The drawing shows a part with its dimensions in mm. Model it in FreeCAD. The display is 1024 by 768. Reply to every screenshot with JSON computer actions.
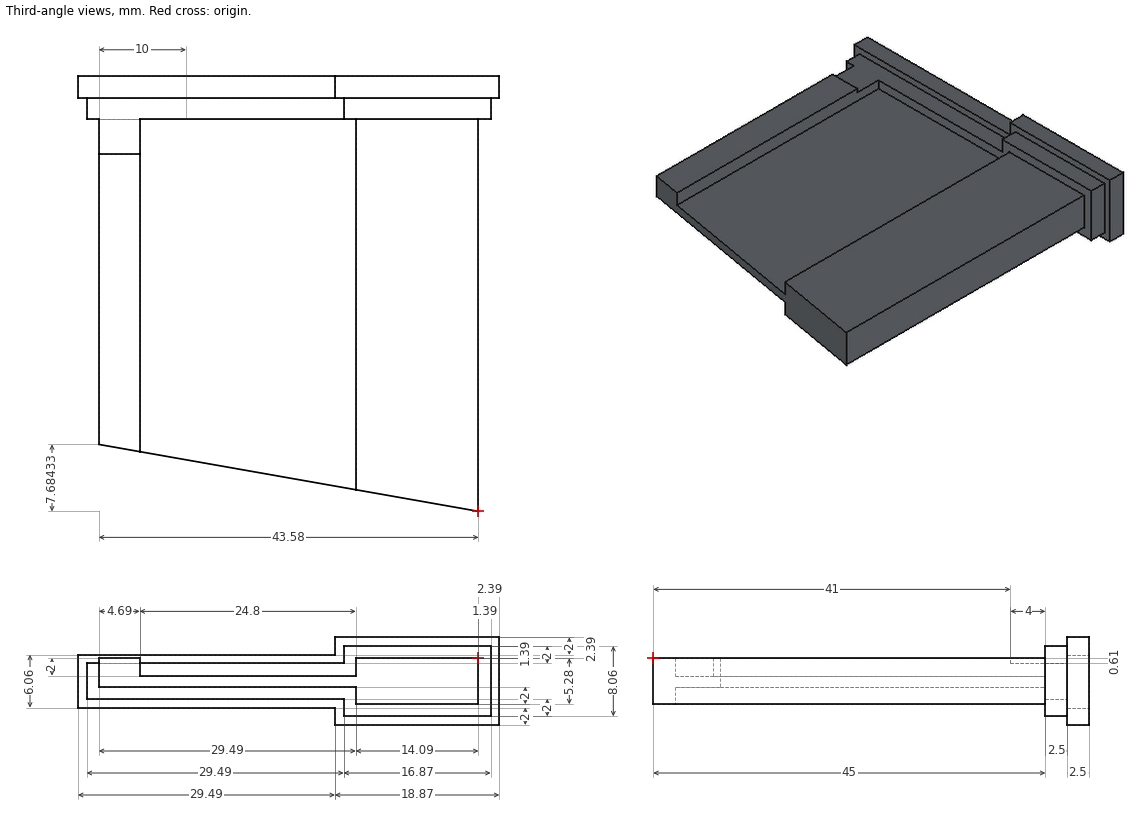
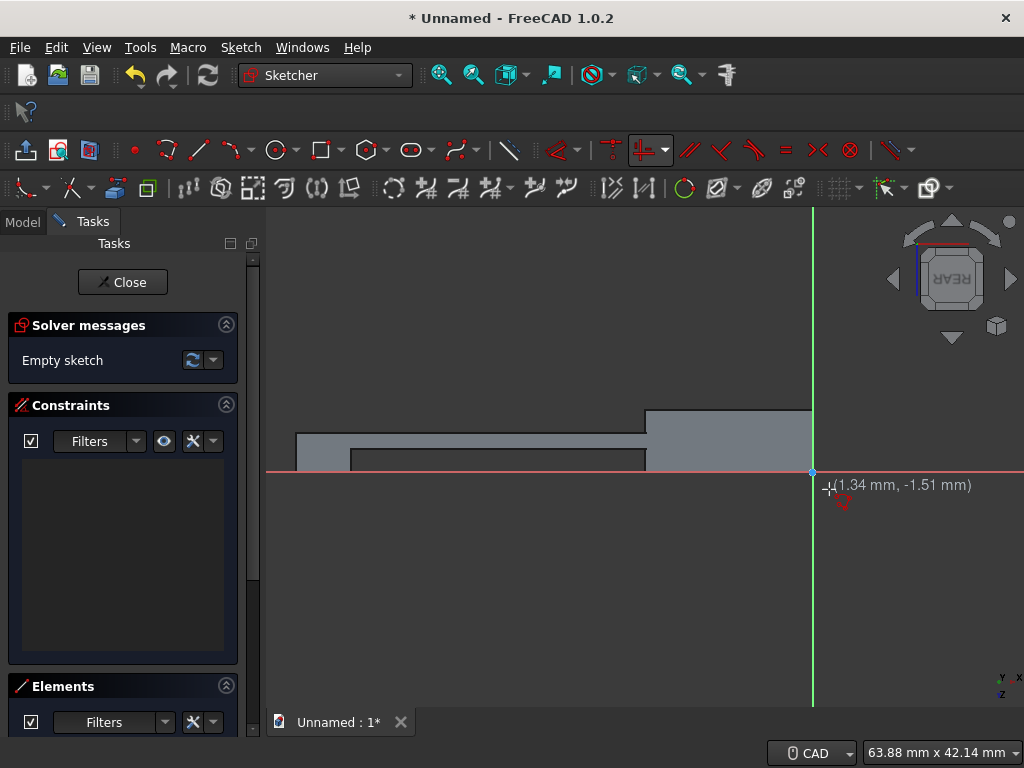
{"action": "left_click", "coordinate": [829, 489]}
{"action": "left_click", "coordinate": [829, 393]}
{"action": "left_click", "coordinate": [629, 393]}
{"action": "left_click", "coordinate": [629, 417]}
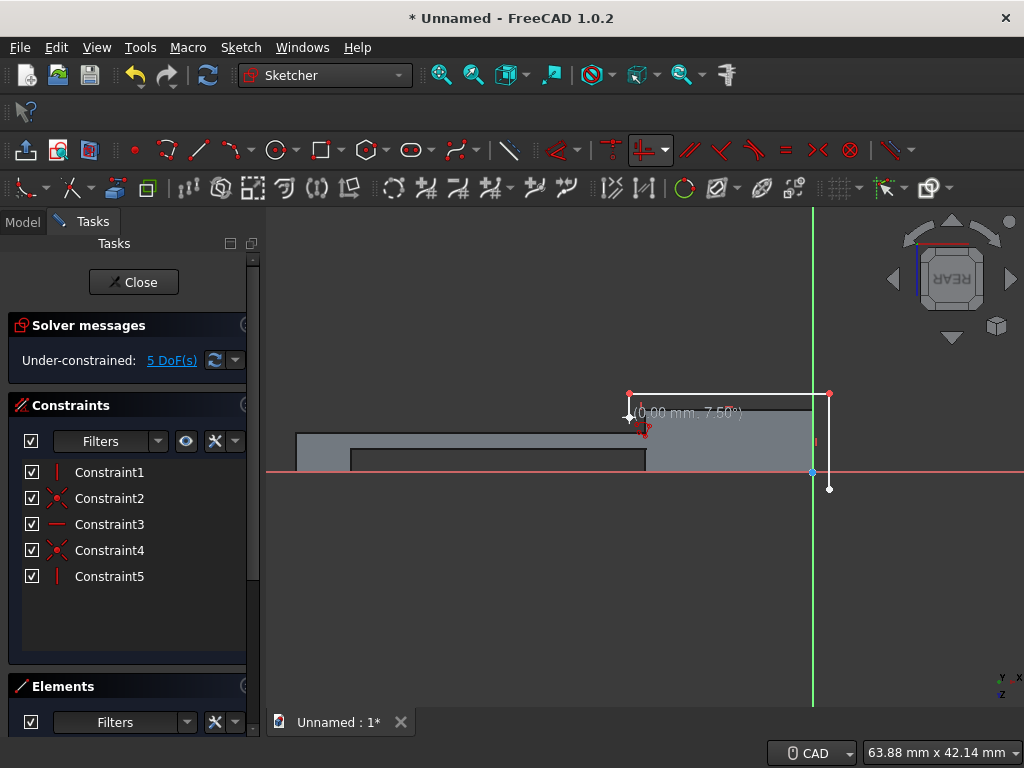
{"action": "scroll", "coordinate": [622, 490], "scroll_direction": "down", "scroll_amount": 2}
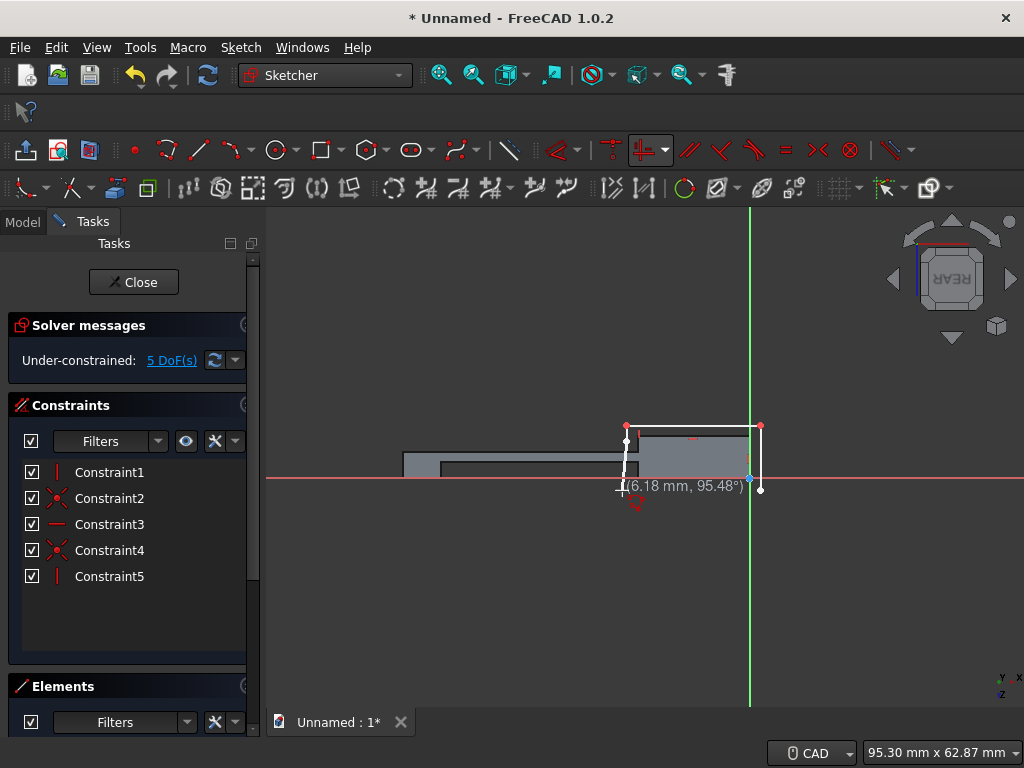
{"action": "left_click", "coordinate": [392, 441]}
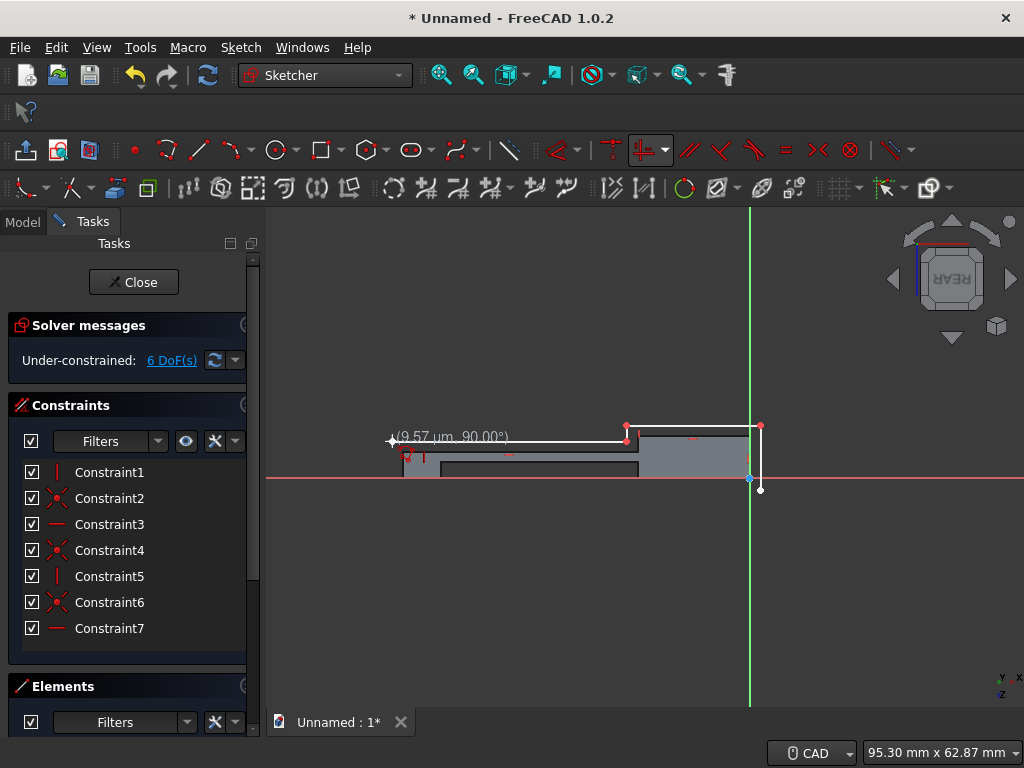
{"action": "scroll", "coordinate": [392, 473], "scroll_direction": "up", "scroll_amount": 6}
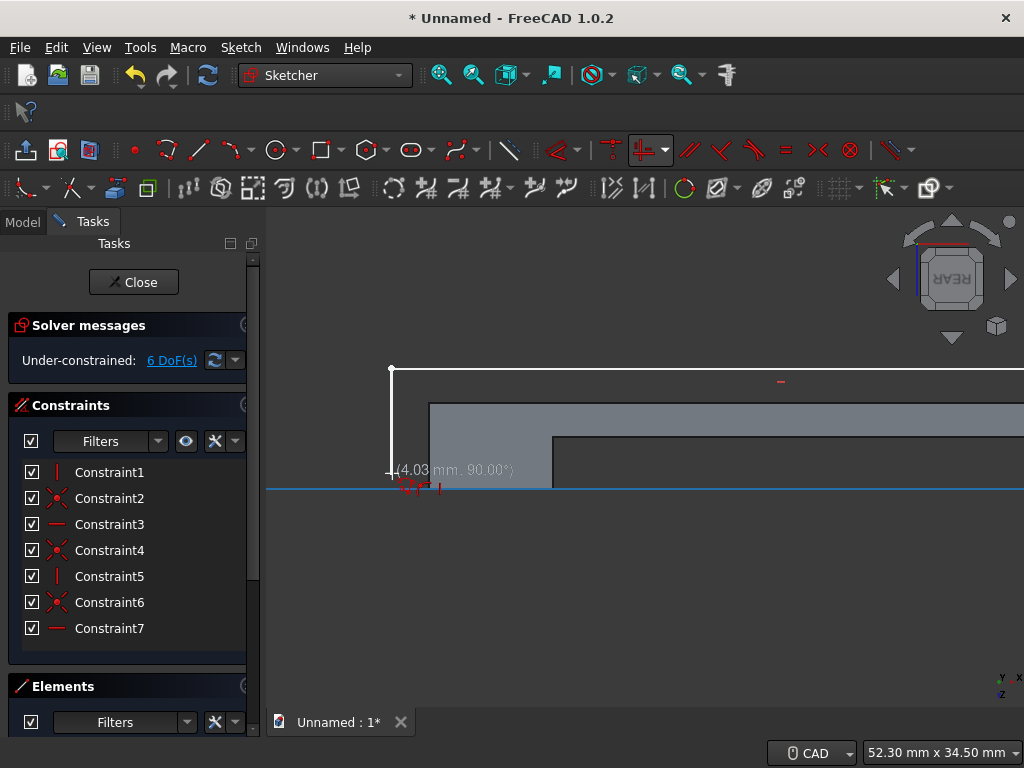
{"action": "left_click", "coordinate": [392, 473]}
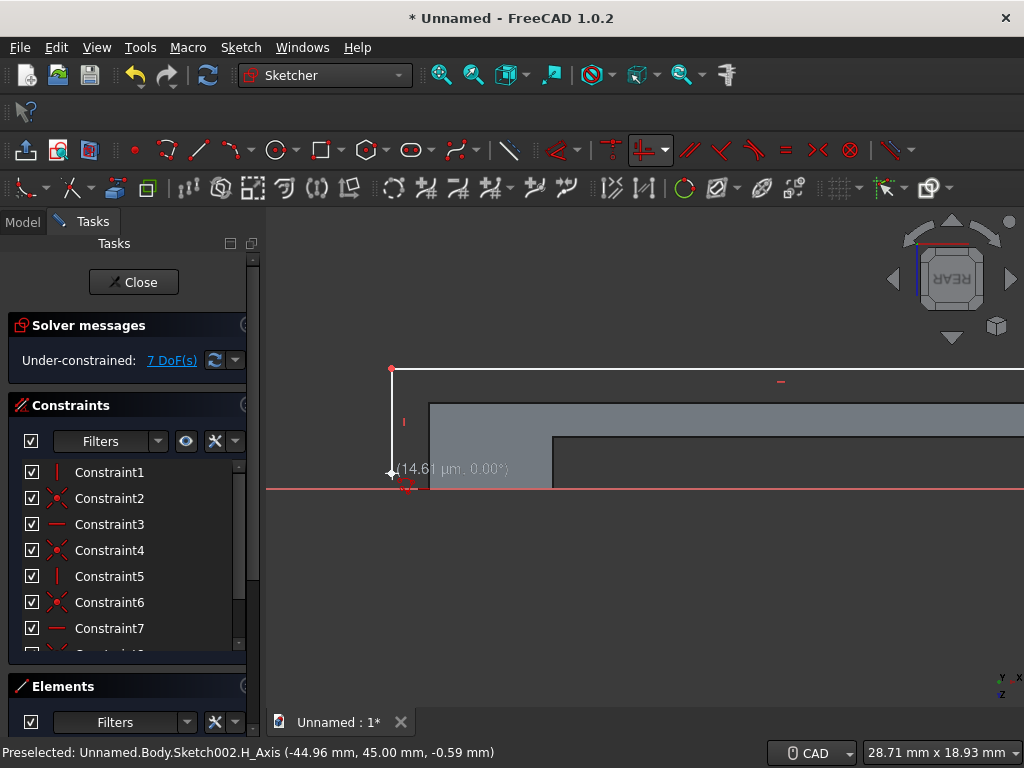
{"action": "scroll", "coordinate": [392, 473], "scroll_direction": "down", "scroll_amount": 6}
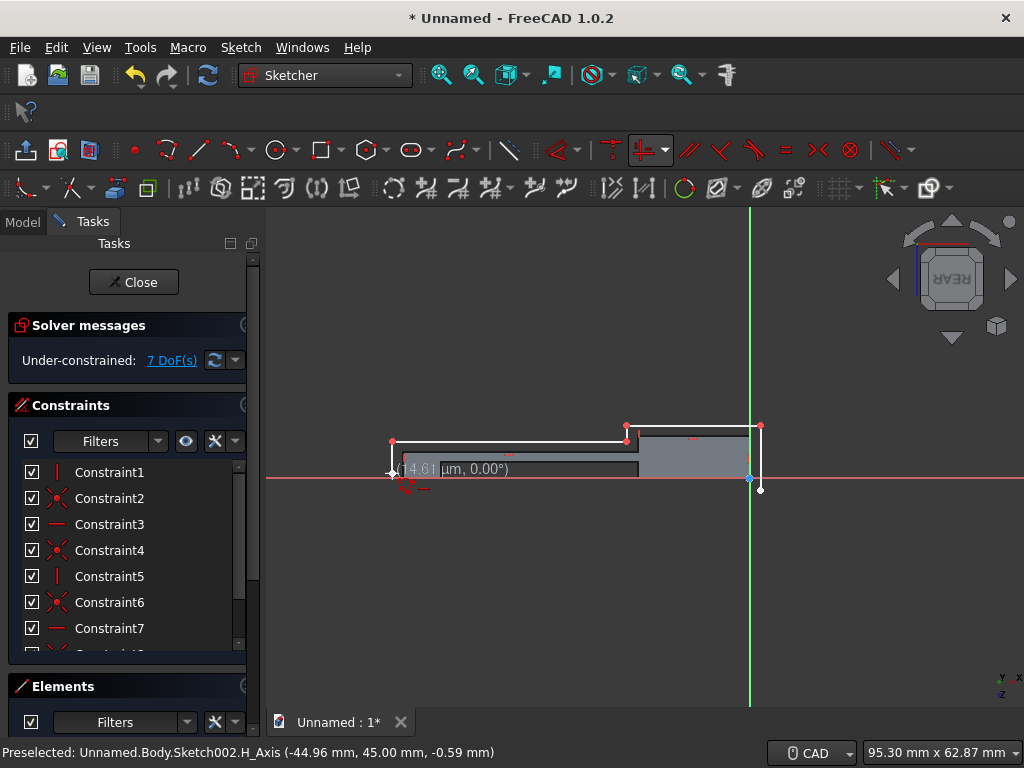
{"action": "scroll", "coordinate": [627, 473], "scroll_direction": "up", "scroll_amount": 6}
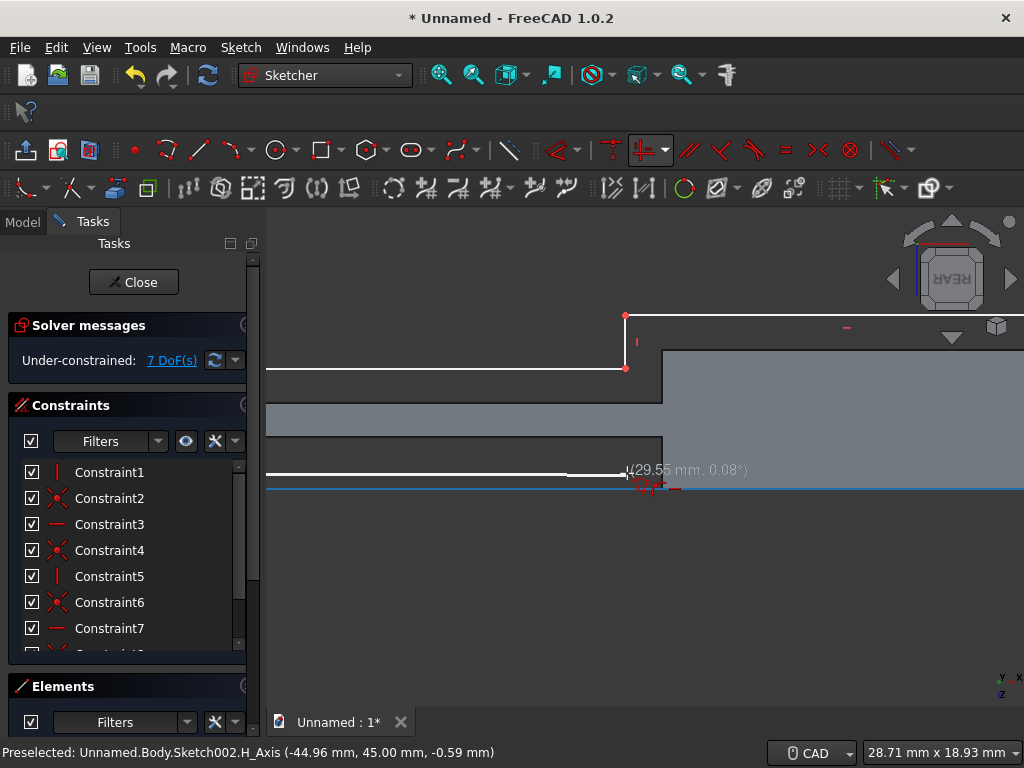
{"action": "left_click", "coordinate": [625, 473]}
{"action": "left_click", "coordinate": [625, 526]}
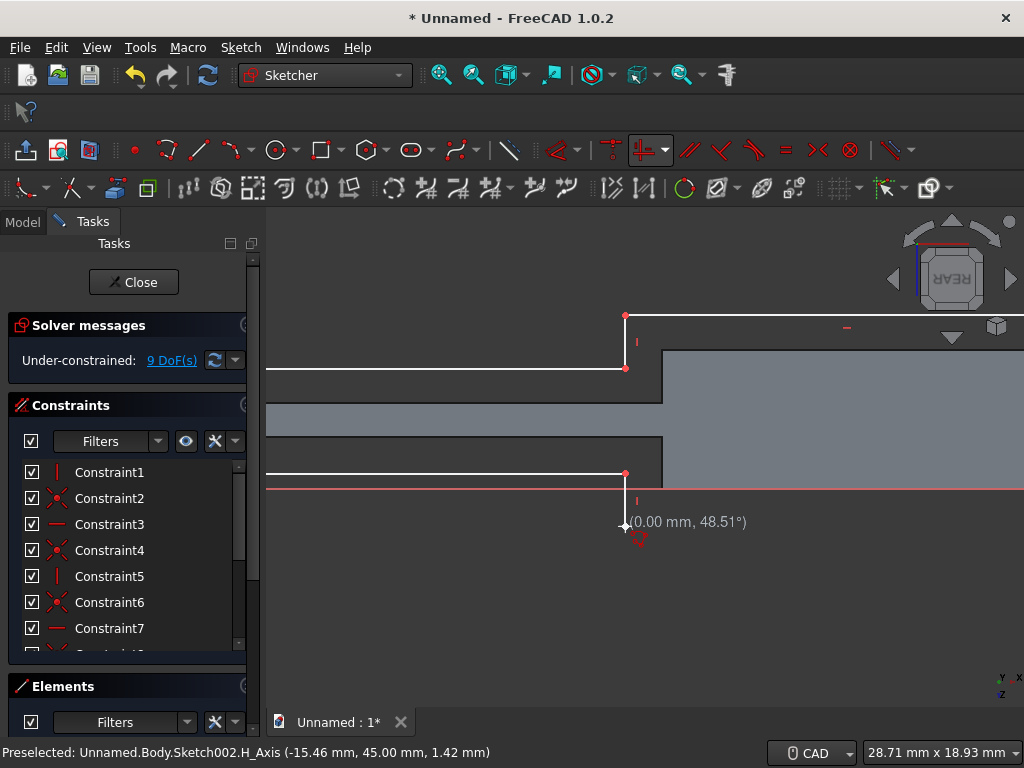
{"action": "scroll", "coordinate": [627, 473], "scroll_direction": "down", "scroll_amount": 6}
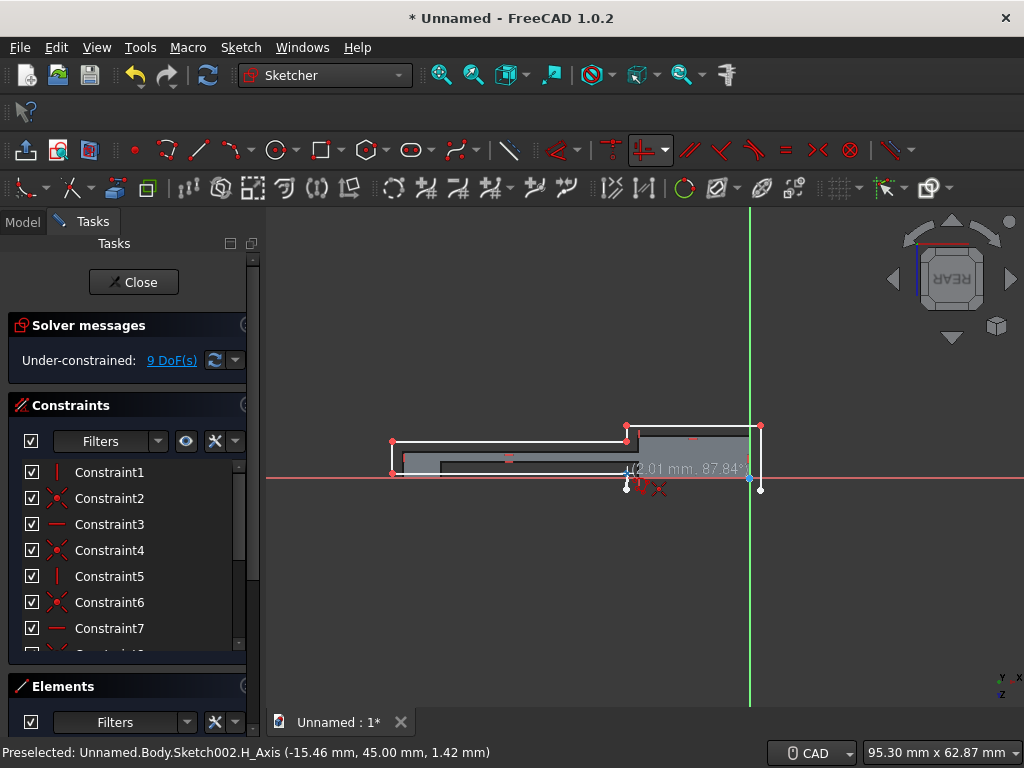
{"action": "scroll", "coordinate": [761, 489], "scroll_direction": "up", "scroll_amount": 2}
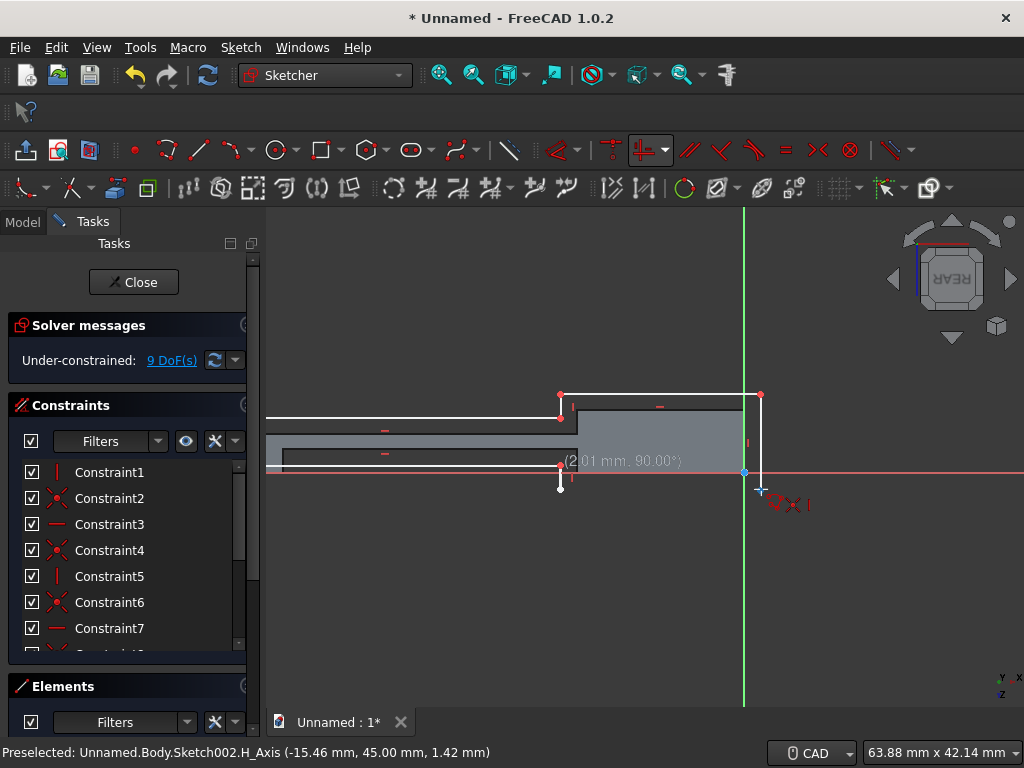
{"action": "left_click", "coordinate": [761, 490]}
{"action": "key", "text": "Escape"}
{"action": "key", "text": "Escape"}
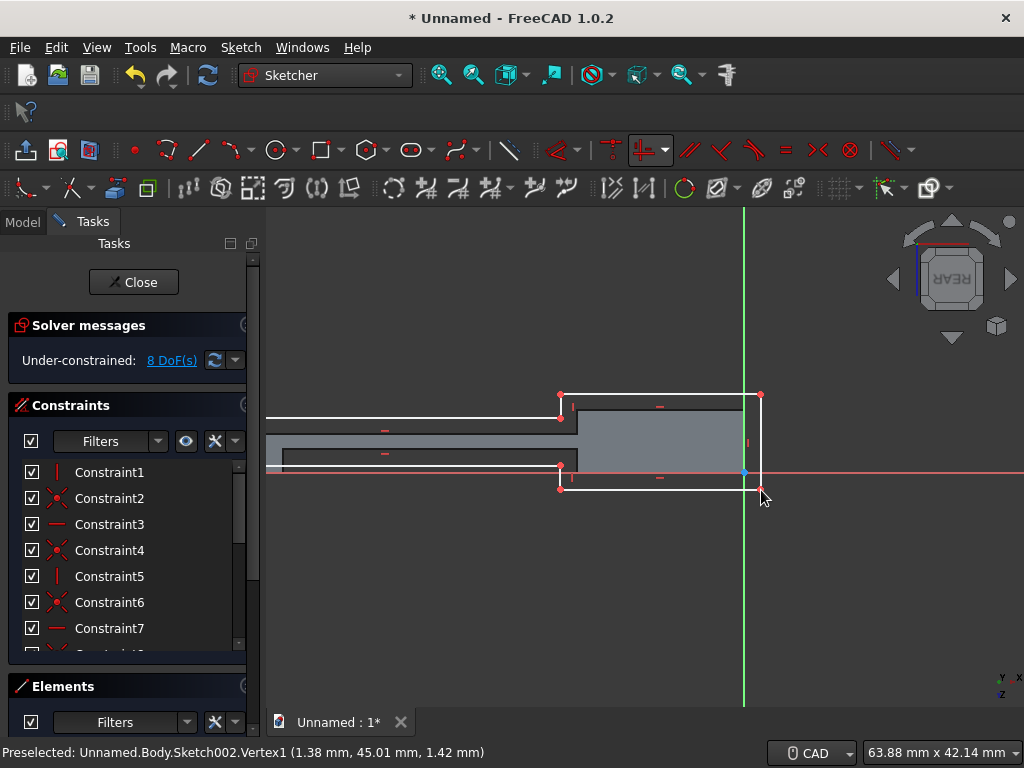
{"action": "left_click", "coordinate": [556, 150]}